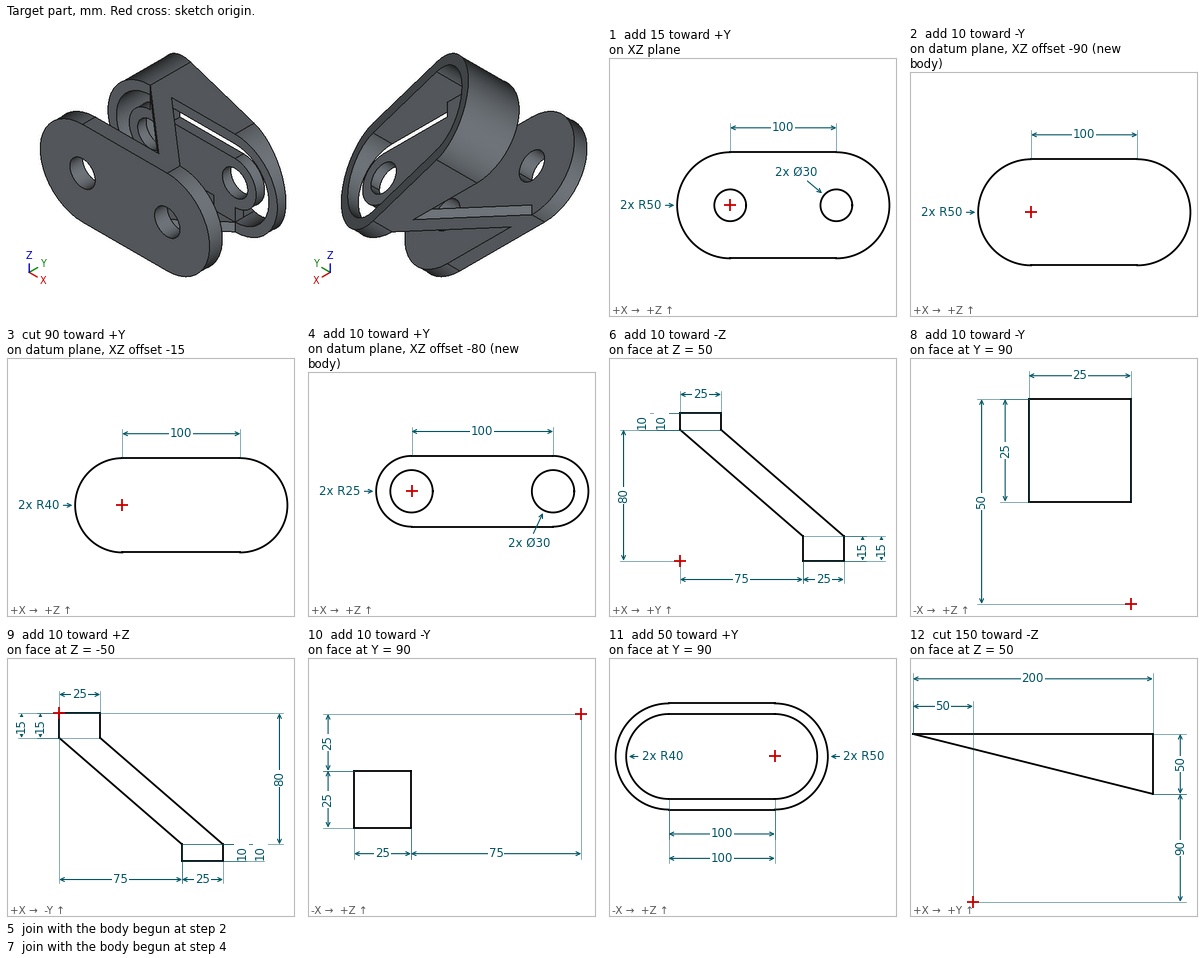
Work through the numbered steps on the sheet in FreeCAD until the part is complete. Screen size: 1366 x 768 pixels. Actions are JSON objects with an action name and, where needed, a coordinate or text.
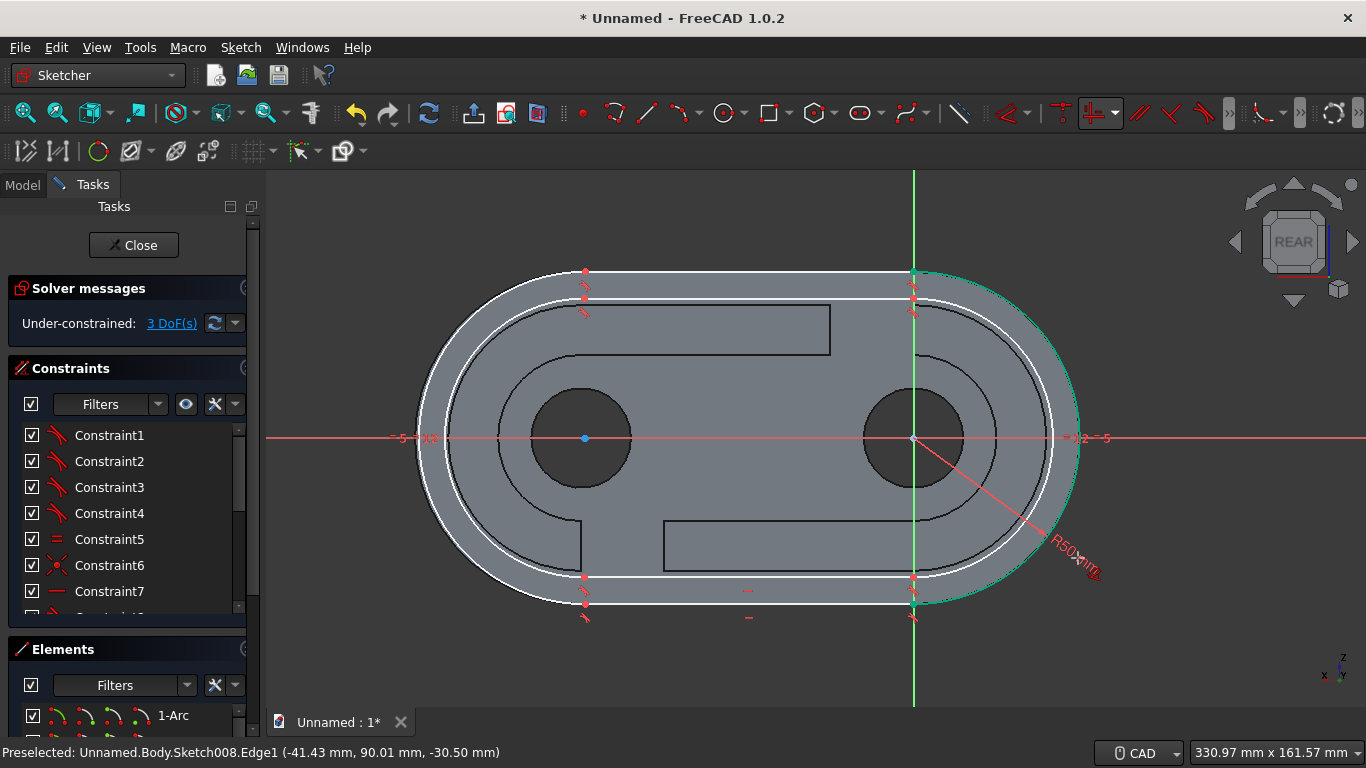
{"action": "left_click", "coordinate": [1026, 520]}
{"action": "left_click", "coordinate": [775, 337]}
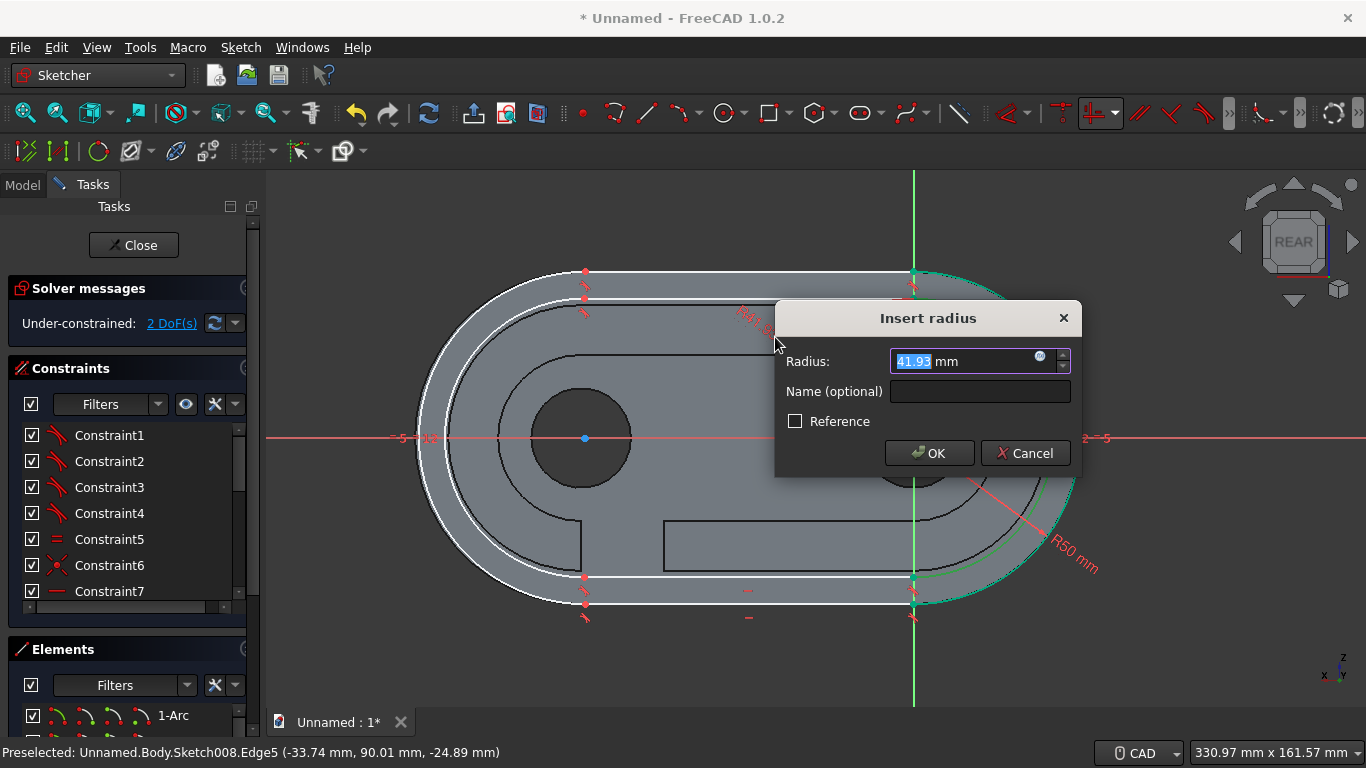
{"action": "type", "text": "40"}
{"action": "key", "text": "Return"}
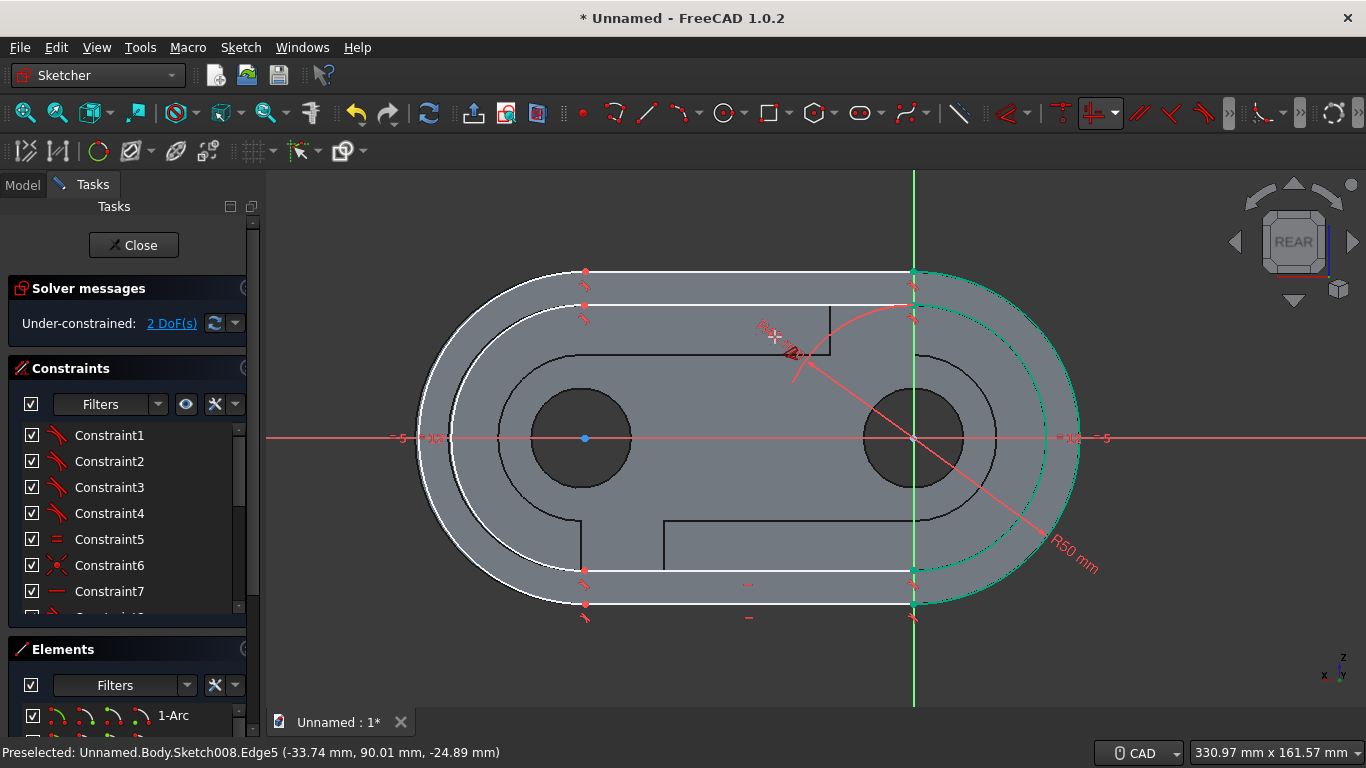
{"action": "left_click", "coordinate": [815, 604]}
{"action": "left_click", "coordinate": [749, 638]}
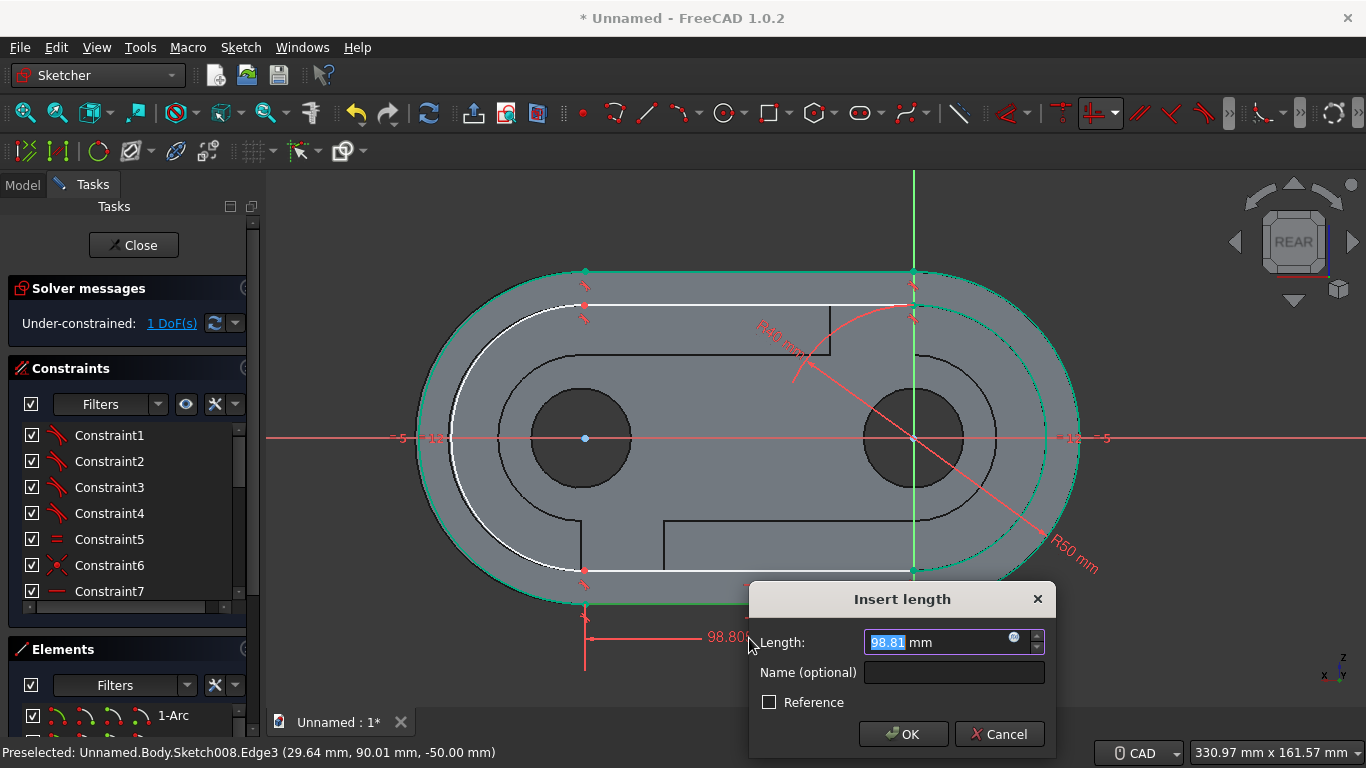
{"action": "type", "text": "100"}
{"action": "key", "text": "Return"}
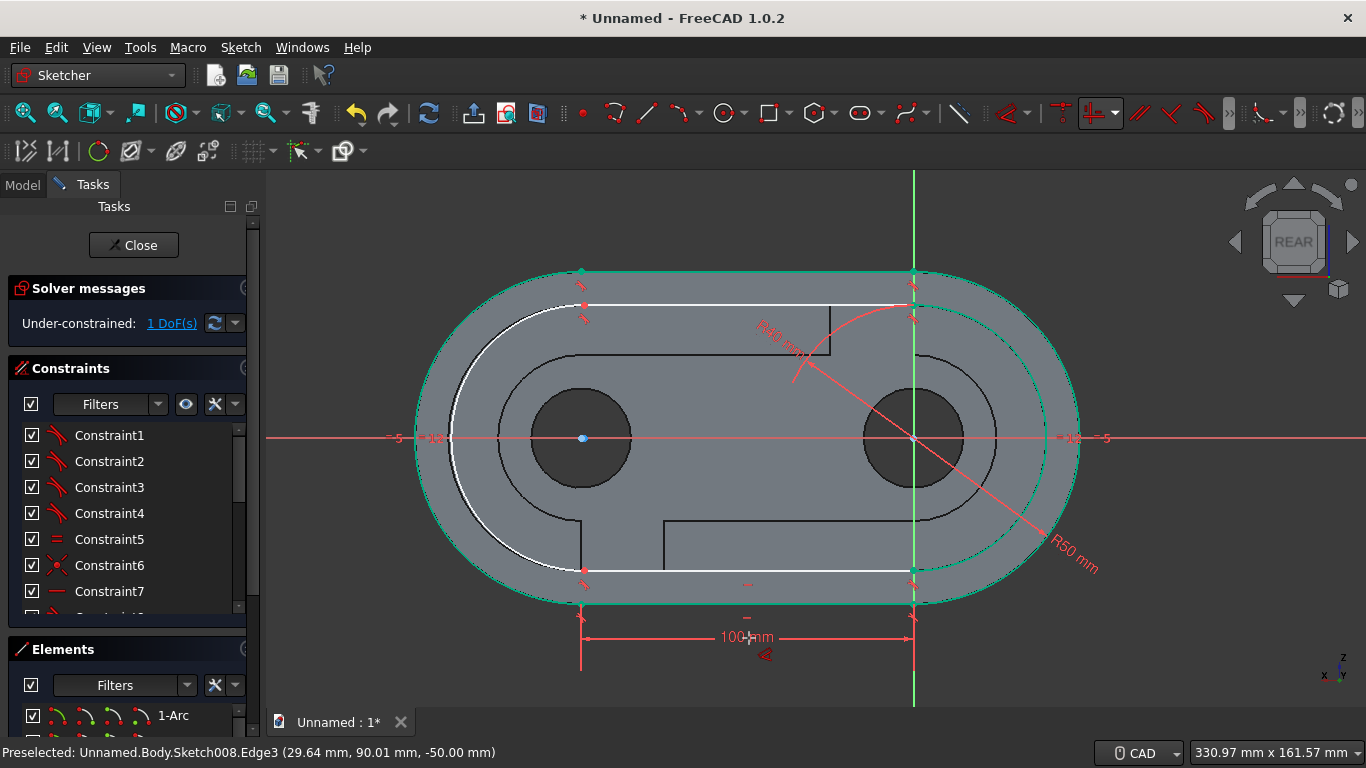
{"action": "left_click", "coordinate": [815, 571]}
{"action": "left_click", "coordinate": [749, 537]}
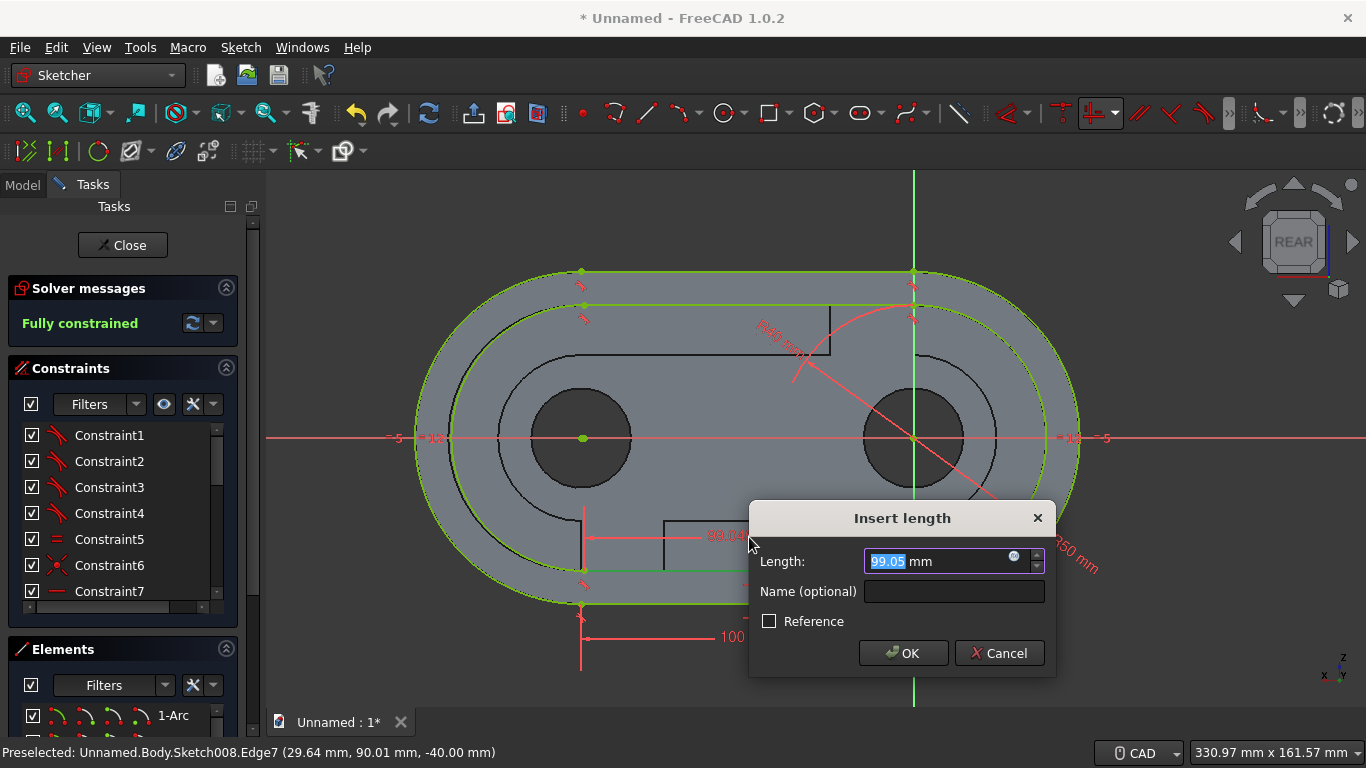
{"action": "type", "text": "100"}
{"action": "key", "text": "Return"}
{"action": "key", "text": "Escape"}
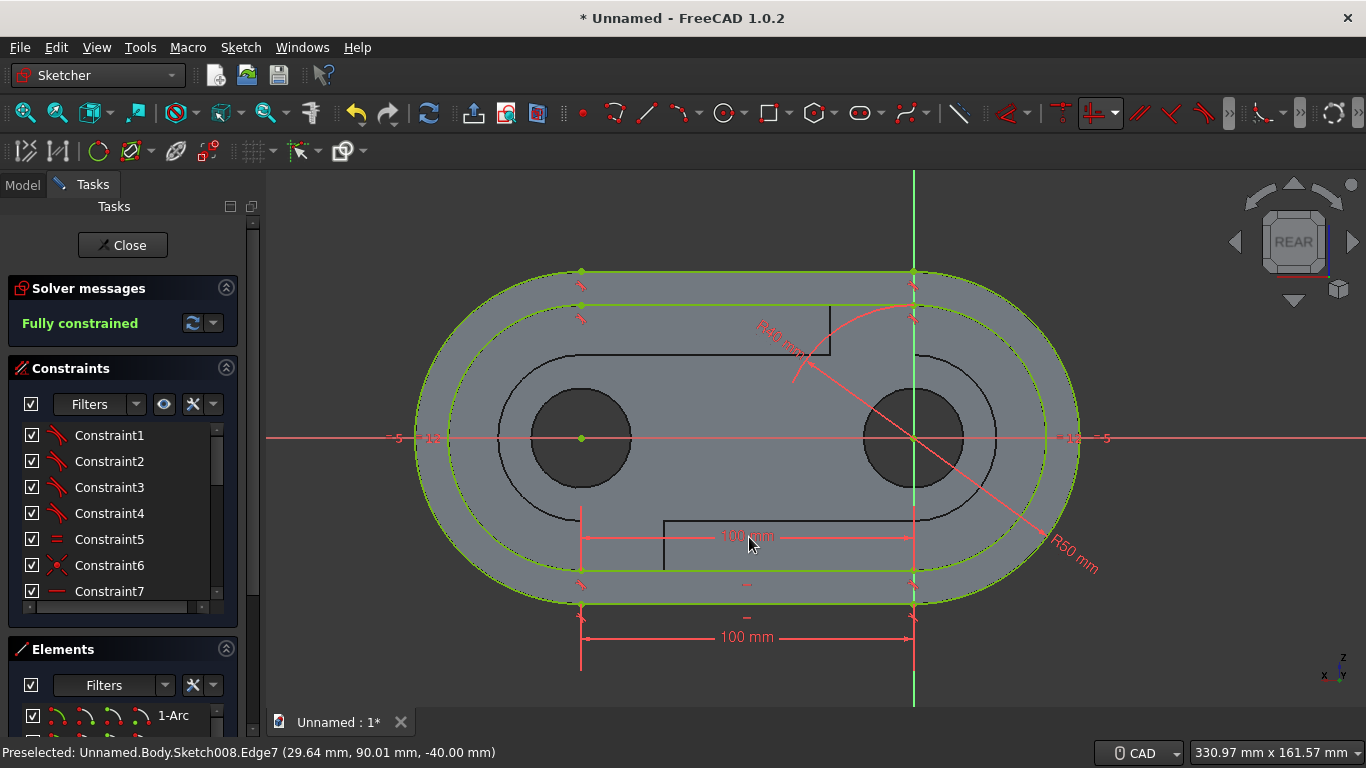
{"action": "left_click", "coordinate": [123, 245]}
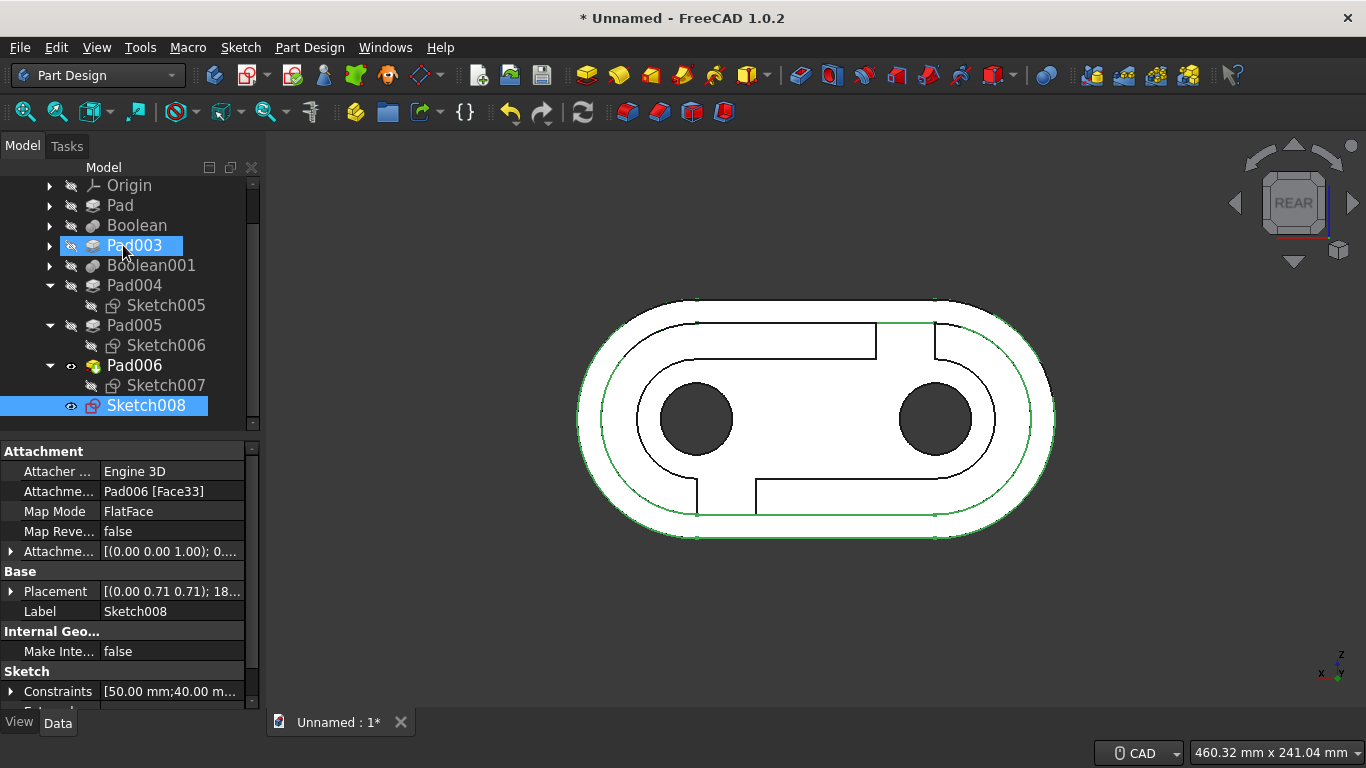
{"action": "left_click", "coordinate": [588, 76]}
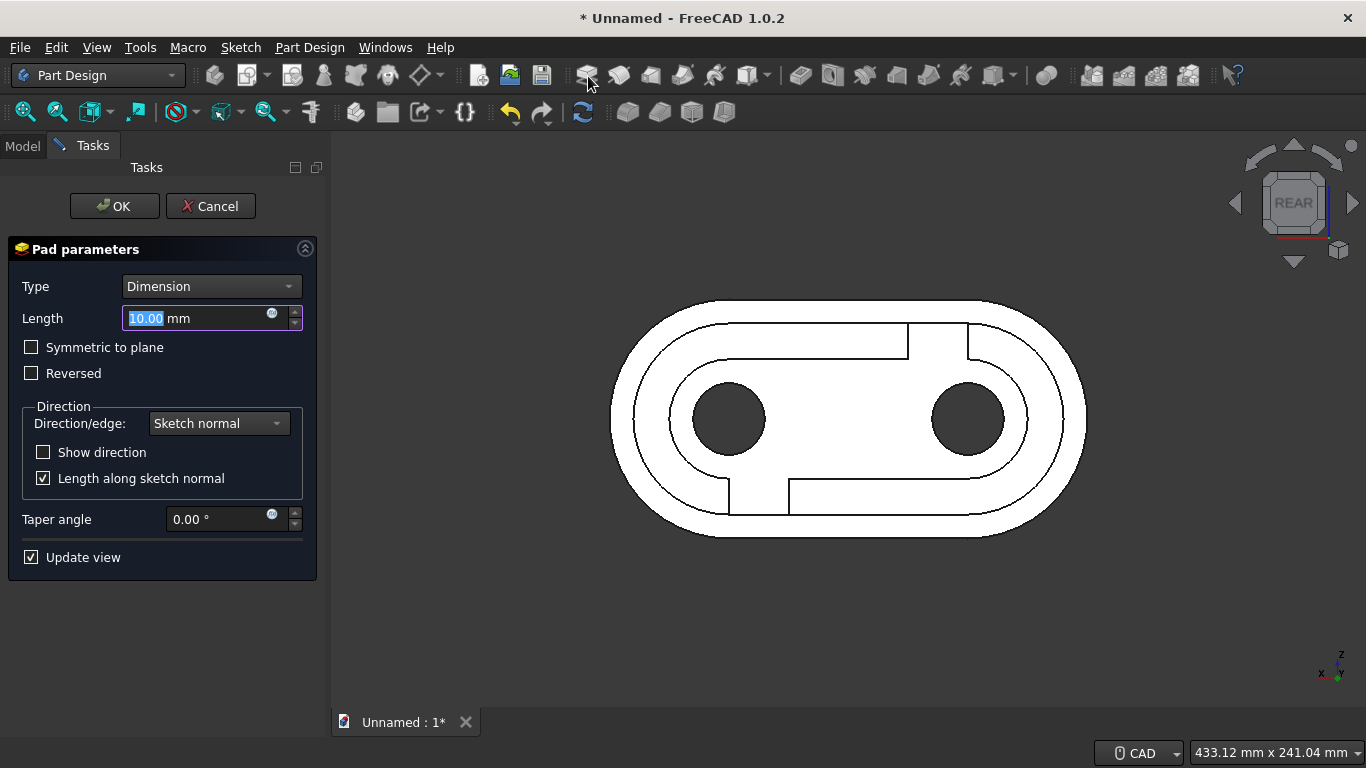
{"action": "type", "text": "50"}
{"action": "key", "text": "Tab"}